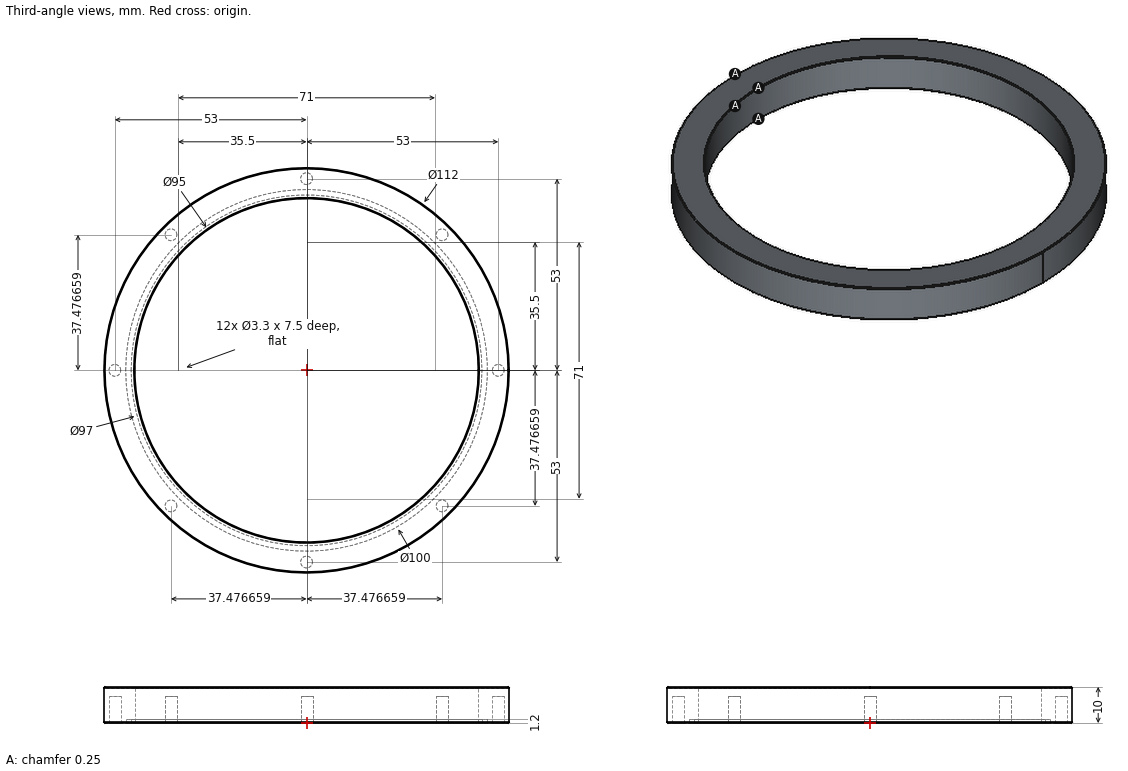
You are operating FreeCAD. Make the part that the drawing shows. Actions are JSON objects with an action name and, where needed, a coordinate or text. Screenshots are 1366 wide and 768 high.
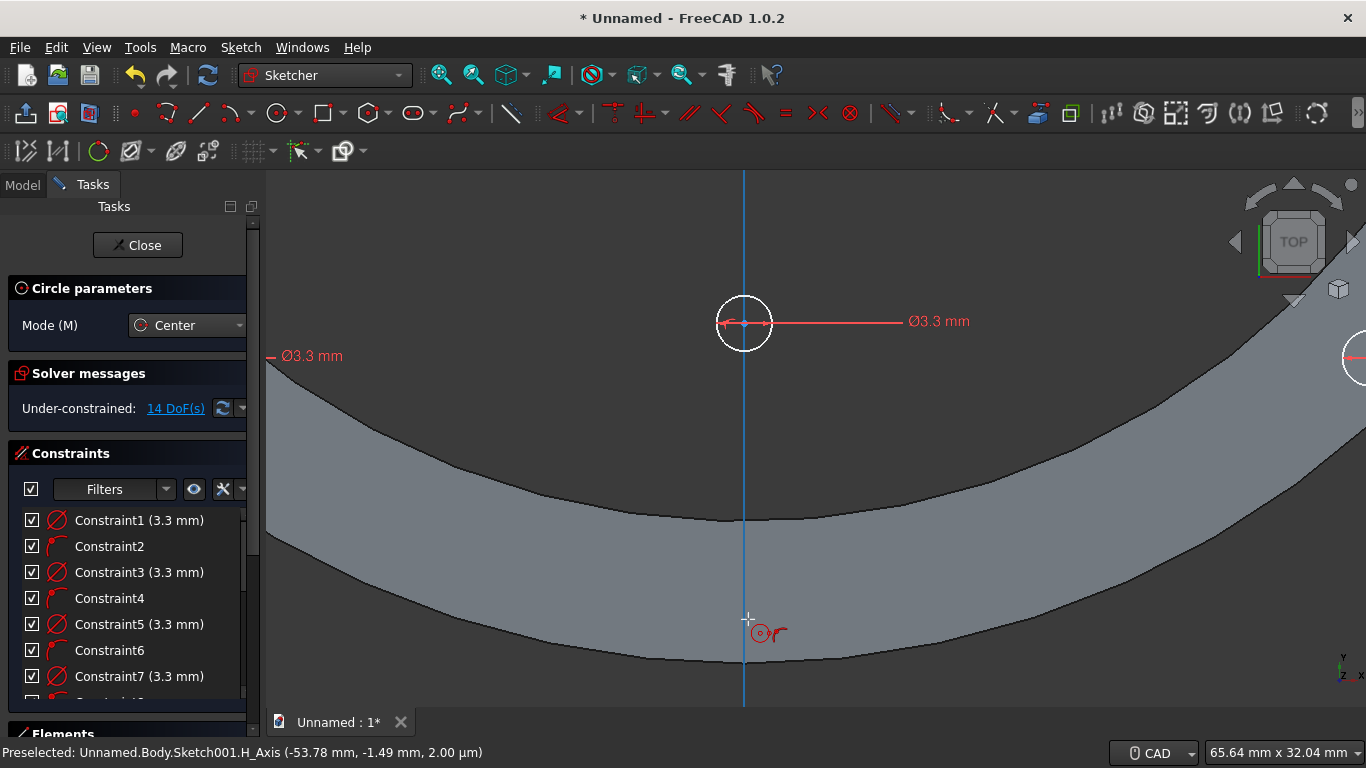
{"action": "scroll", "coordinate": [748, 619], "scroll_direction": "down", "scroll_amount": 8}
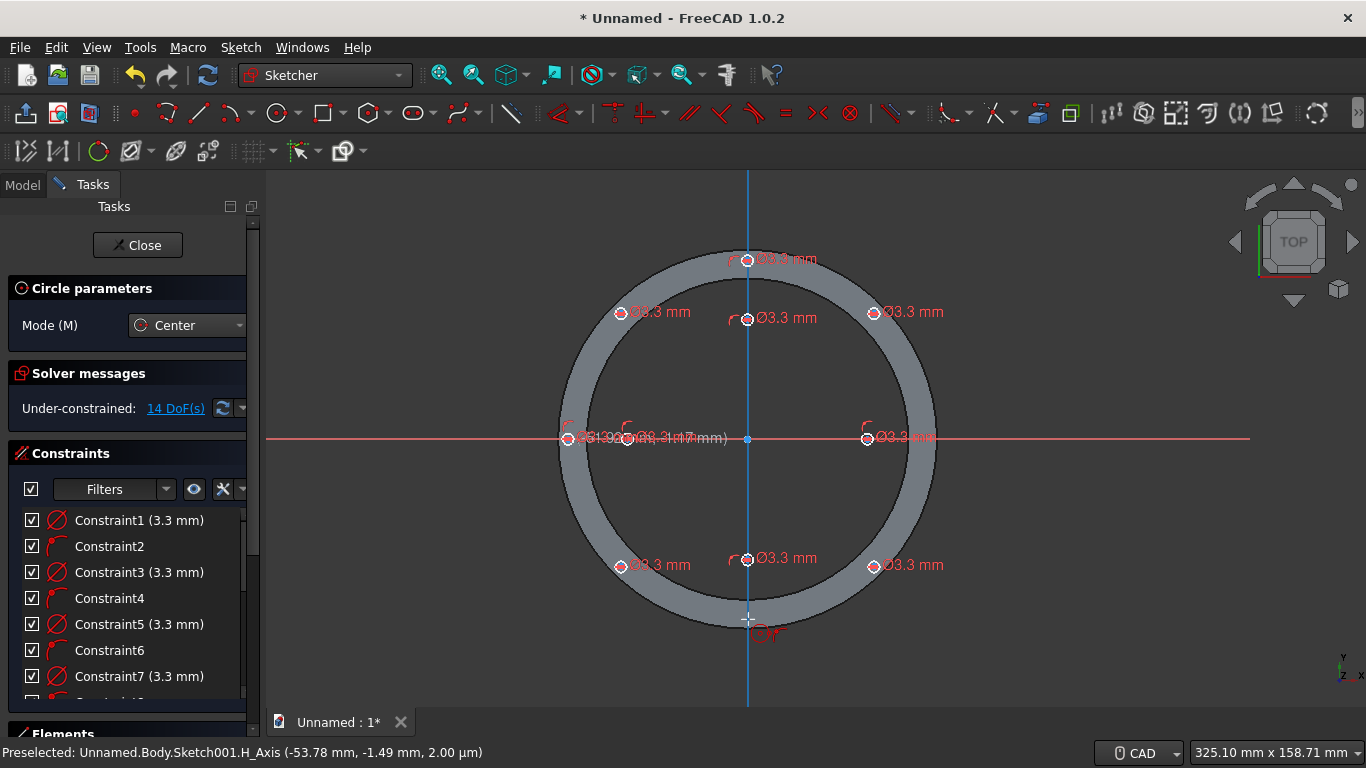
{"action": "left_click", "coordinate": [748, 619]}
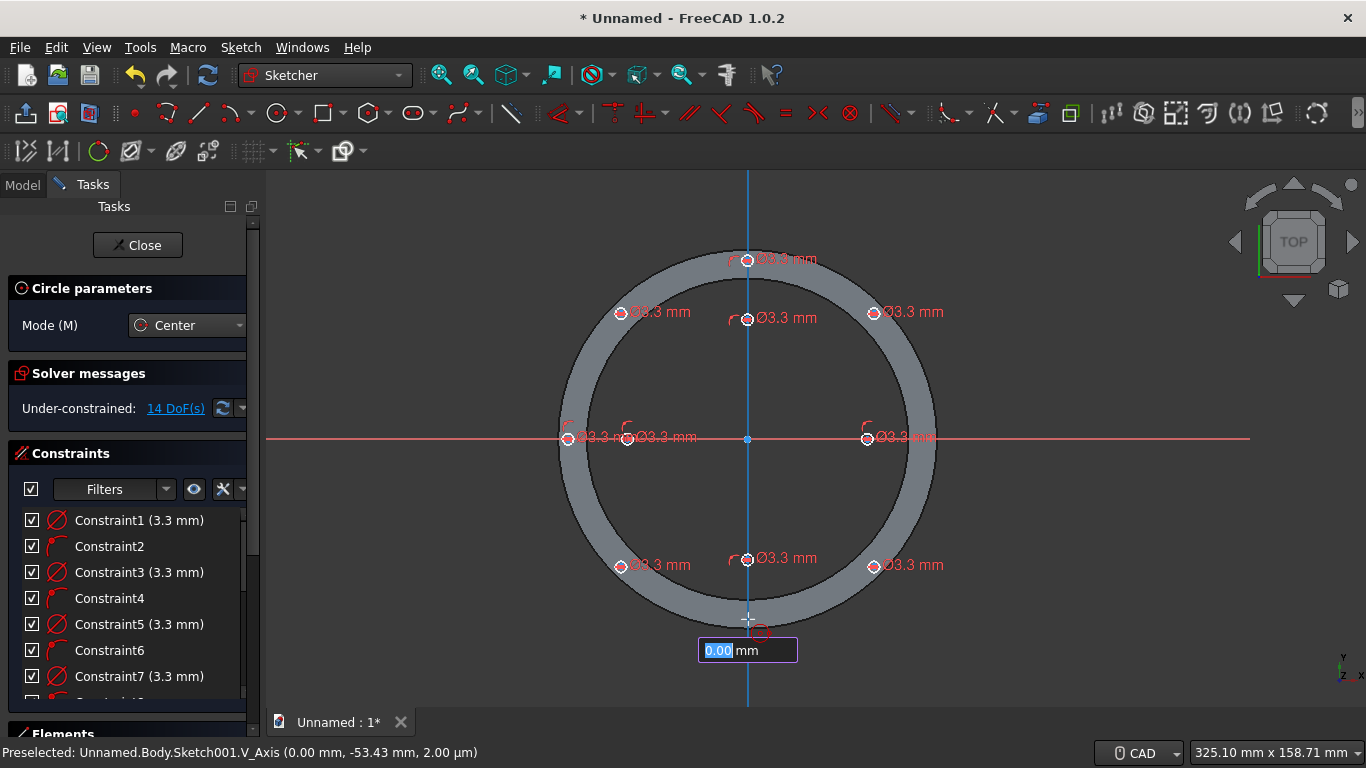
{"action": "scroll", "coordinate": [753, 617], "scroll_direction": "up", "scroll_amount": 6}
{"action": "mouse_move", "coordinate": [751, 614]}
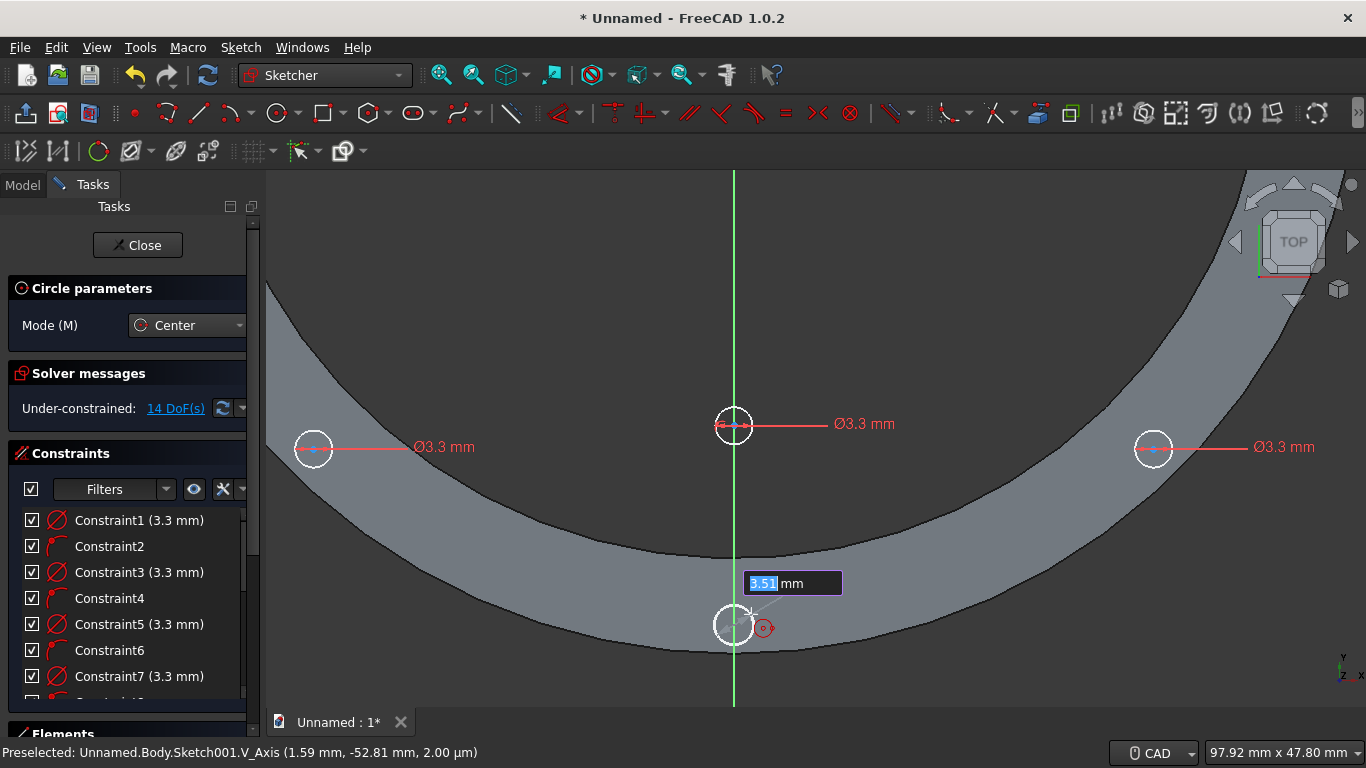
{"action": "type", "text": "3.3"}
{"action": "key", "text": "Return"}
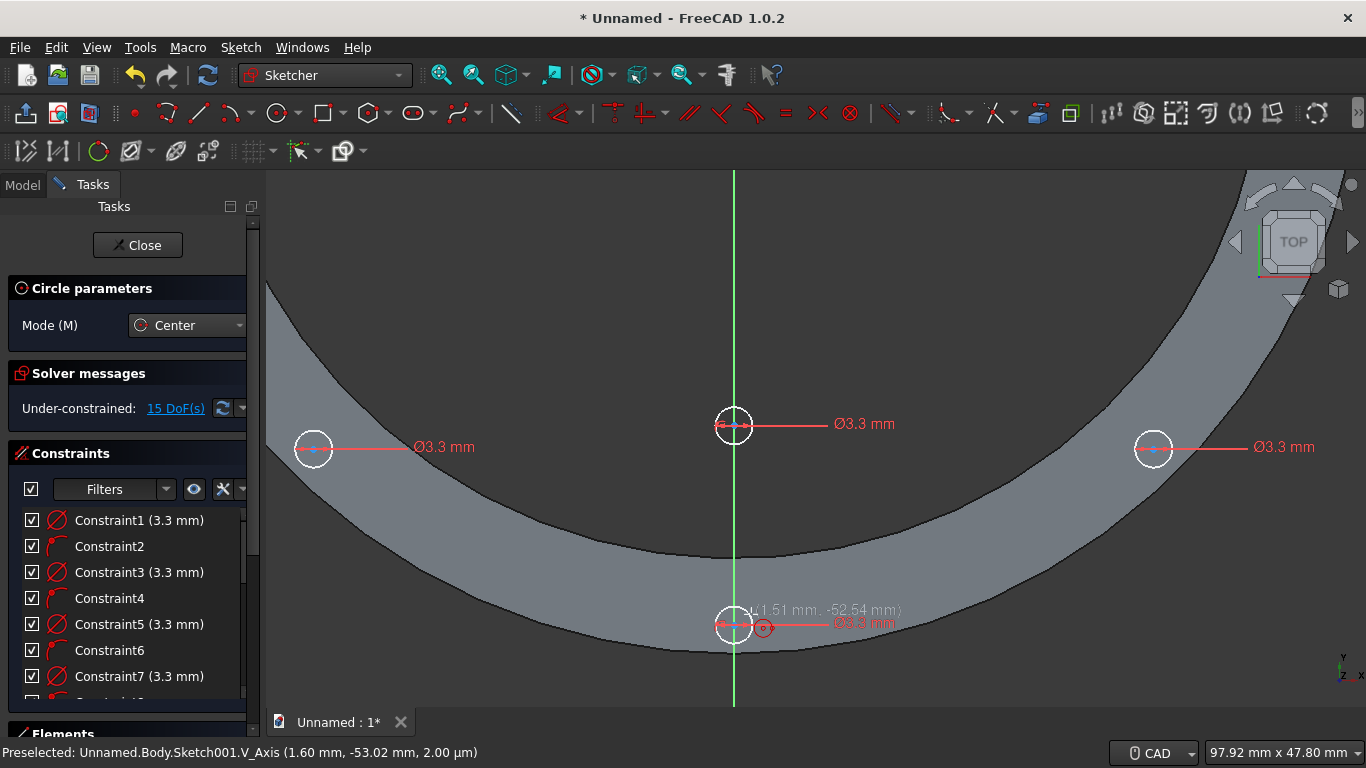
{"action": "scroll", "coordinate": [753, 617], "scroll_direction": "down", "scroll_amount": 6}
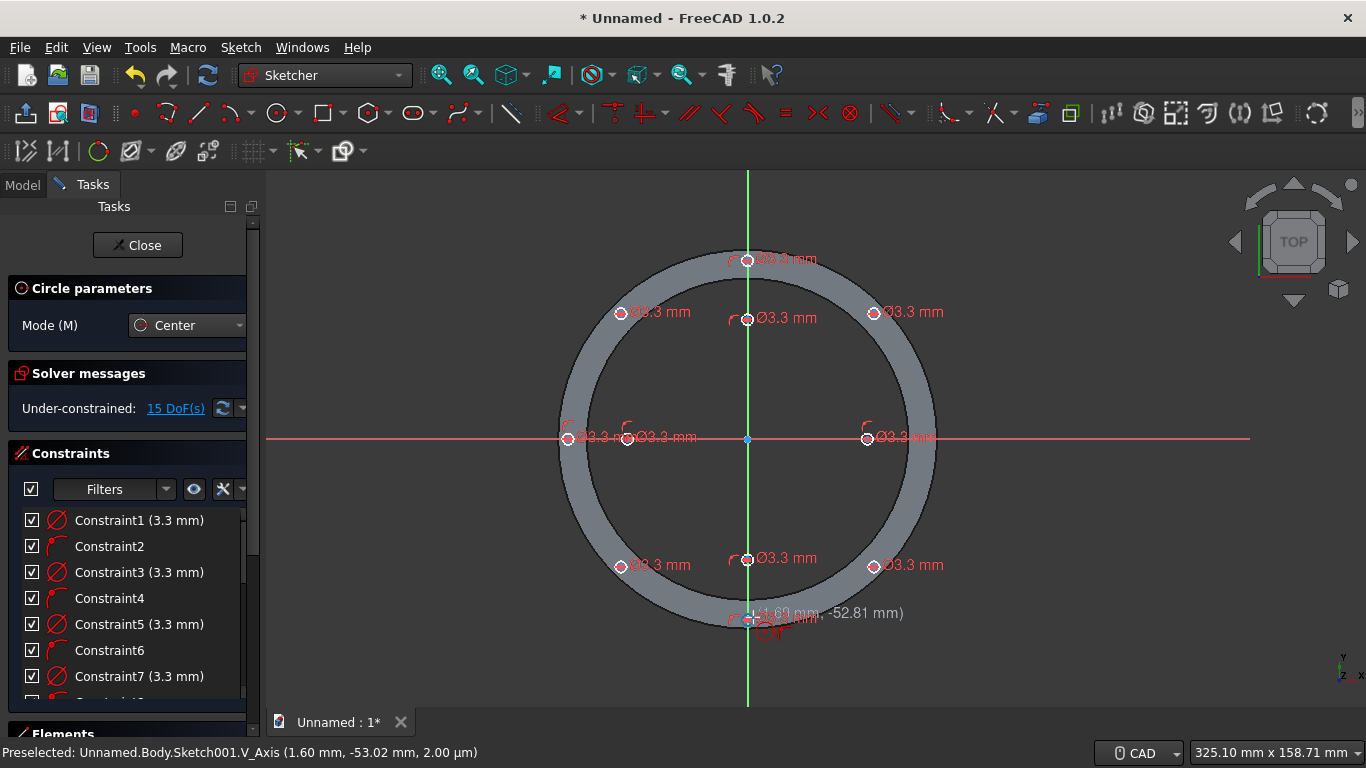
{"action": "scroll", "coordinate": [927, 439], "scroll_direction": "up", "scroll_amount": 8}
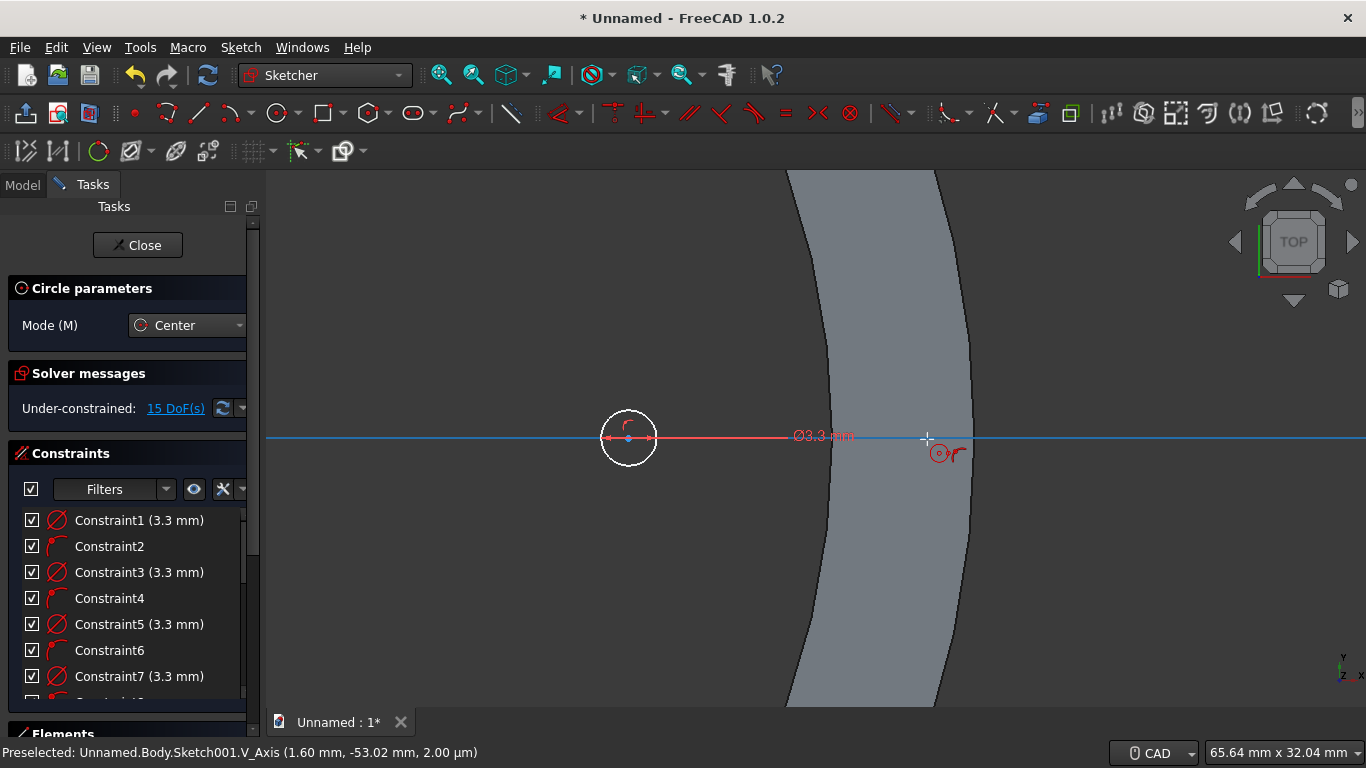
{"action": "scroll", "coordinate": [927, 439], "scroll_direction": "down", "scroll_amount": 8}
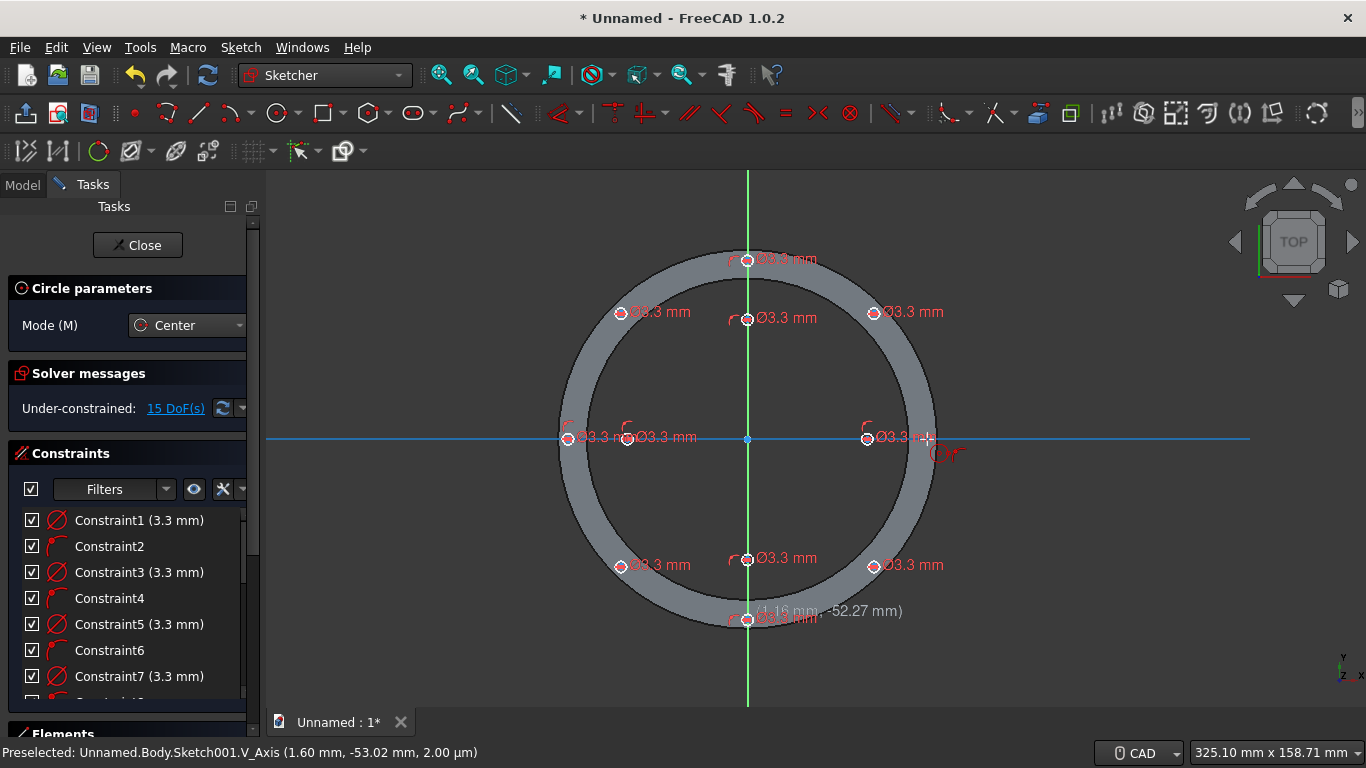
{"action": "left_click", "coordinate": [927, 439]}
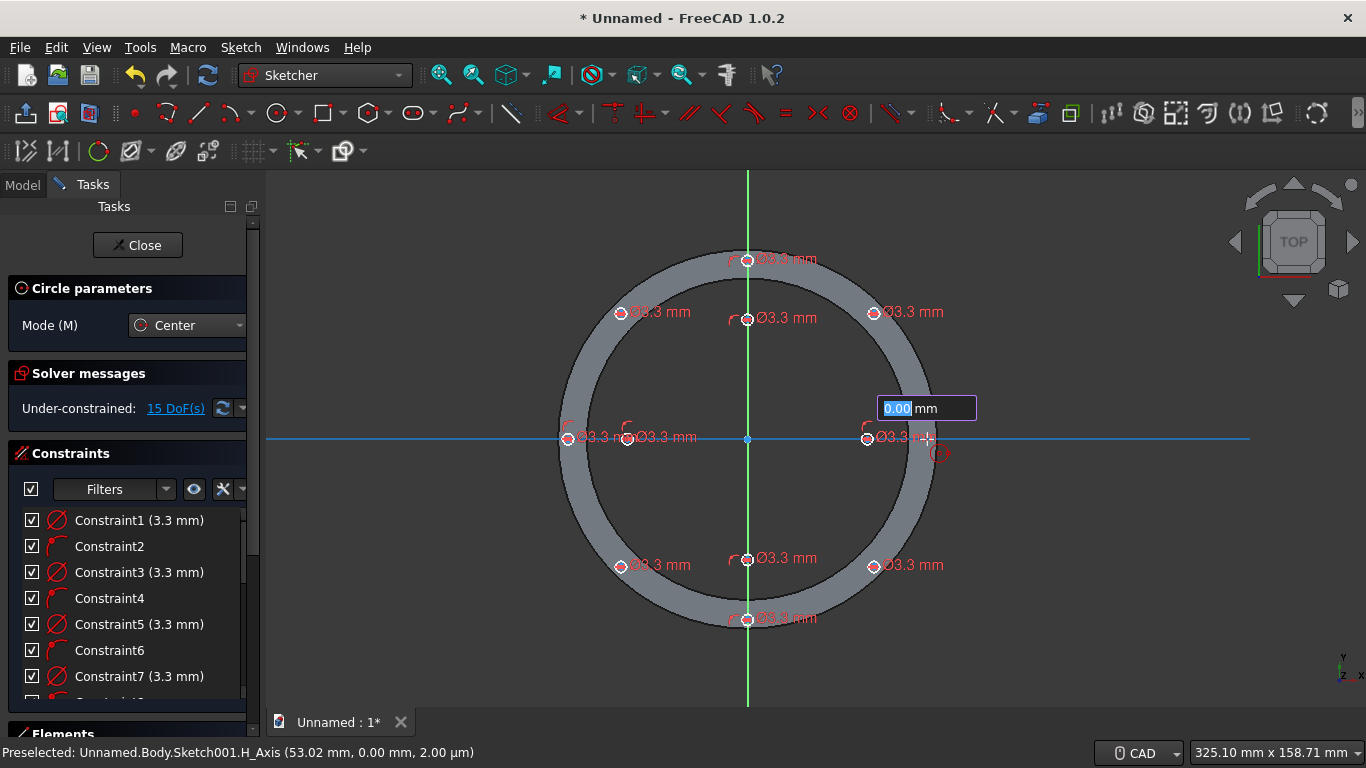
{"action": "scroll", "coordinate": [925, 444], "scroll_direction": "up", "scroll_amount": 6}
{"action": "mouse_move", "coordinate": [924, 444]}